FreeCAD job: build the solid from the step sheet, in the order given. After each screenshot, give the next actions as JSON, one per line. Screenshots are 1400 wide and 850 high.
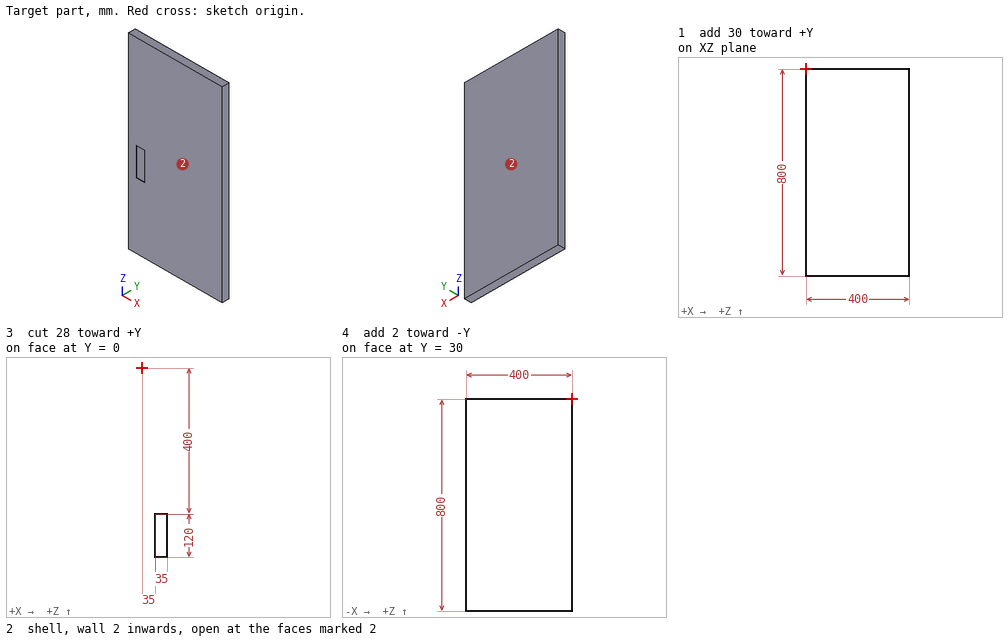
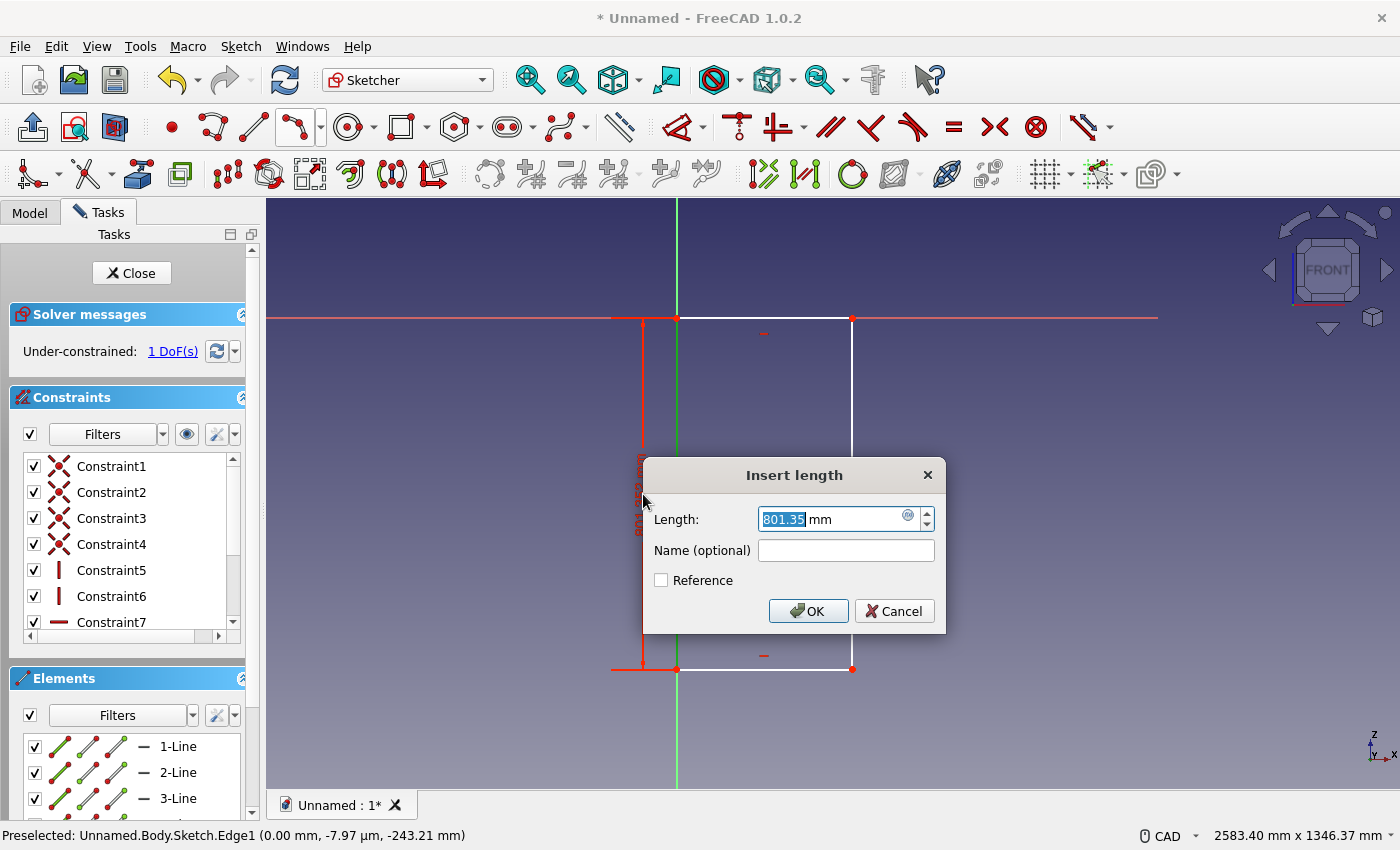
{"action": "type", "text": "800"}
{"action": "key", "text": "Return"}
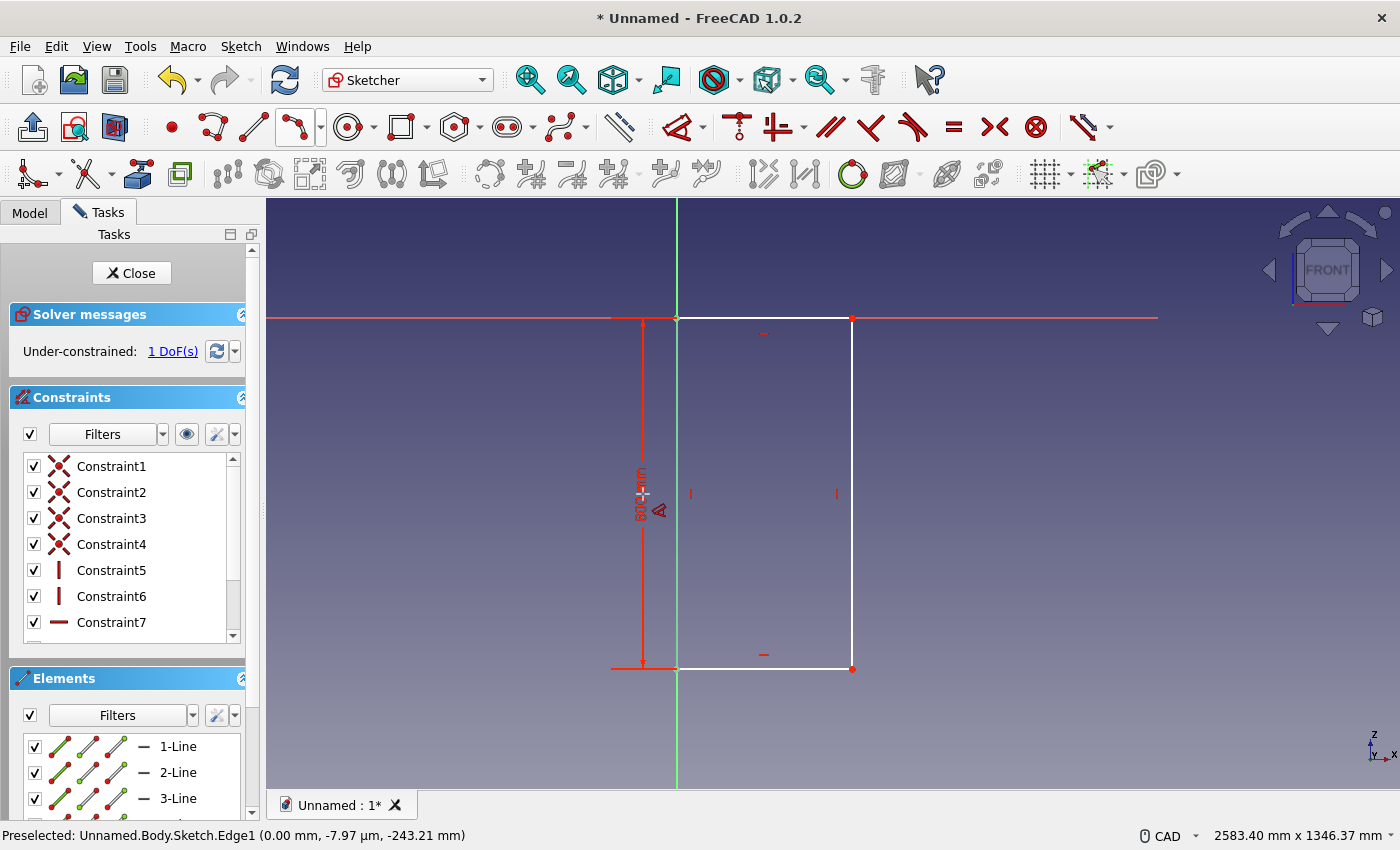
{"action": "left_click", "coordinate": [729, 669]}
{"action": "left_click", "coordinate": [764, 703]}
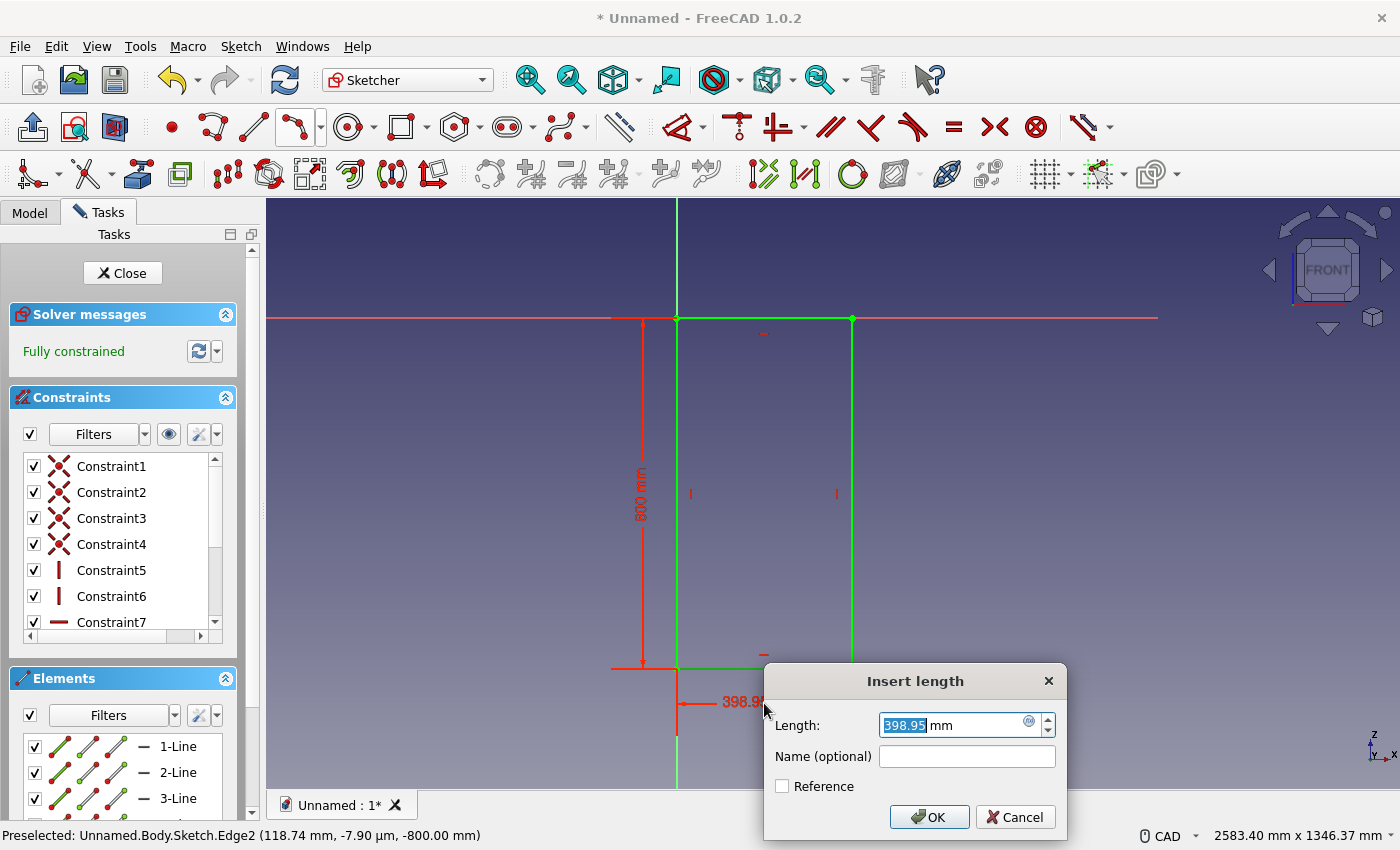
{"action": "type", "text": "400"}
{"action": "key", "text": "Return"}
{"action": "key", "text": "Escape"}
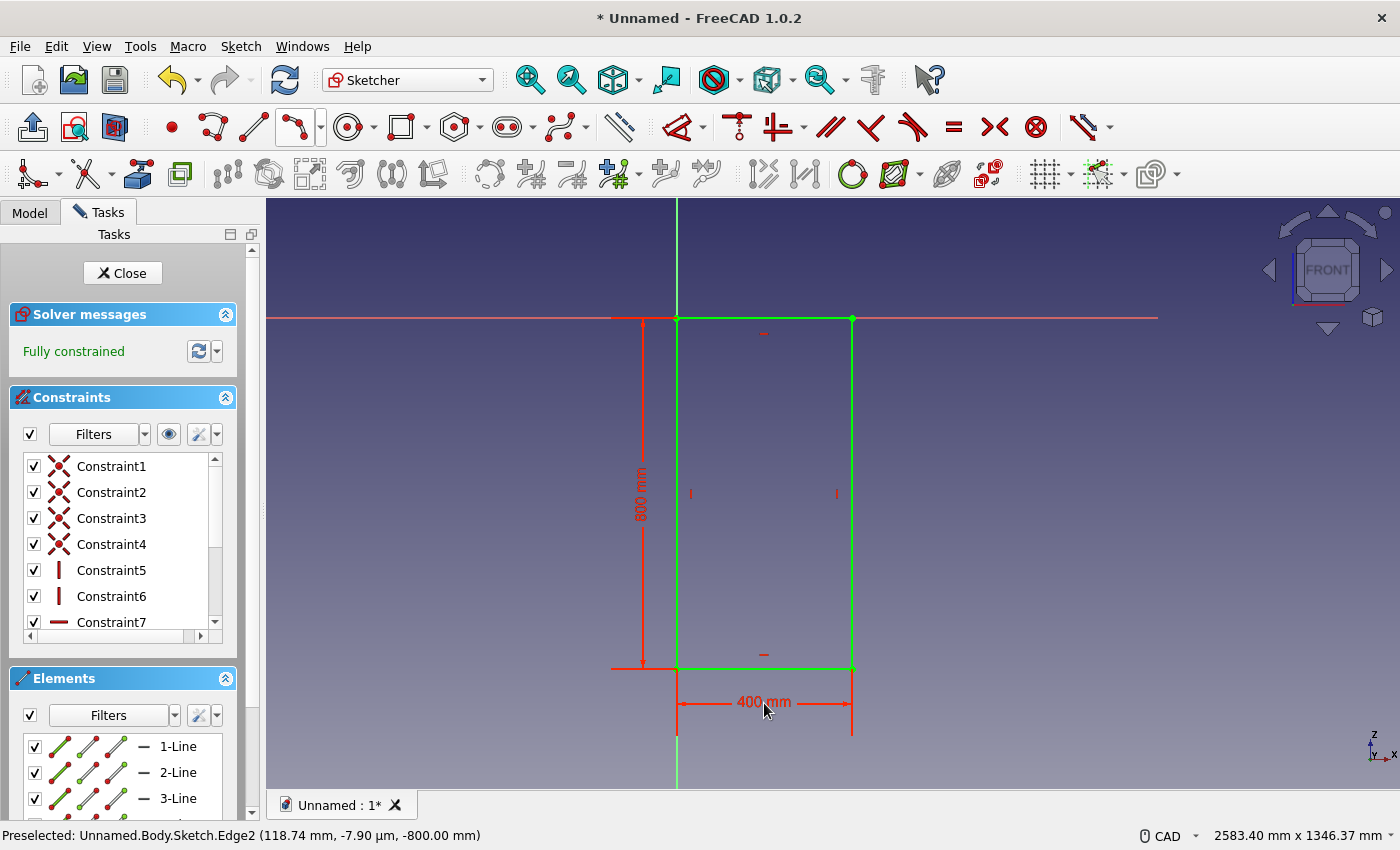
{"action": "left_click", "coordinate": [123, 273]}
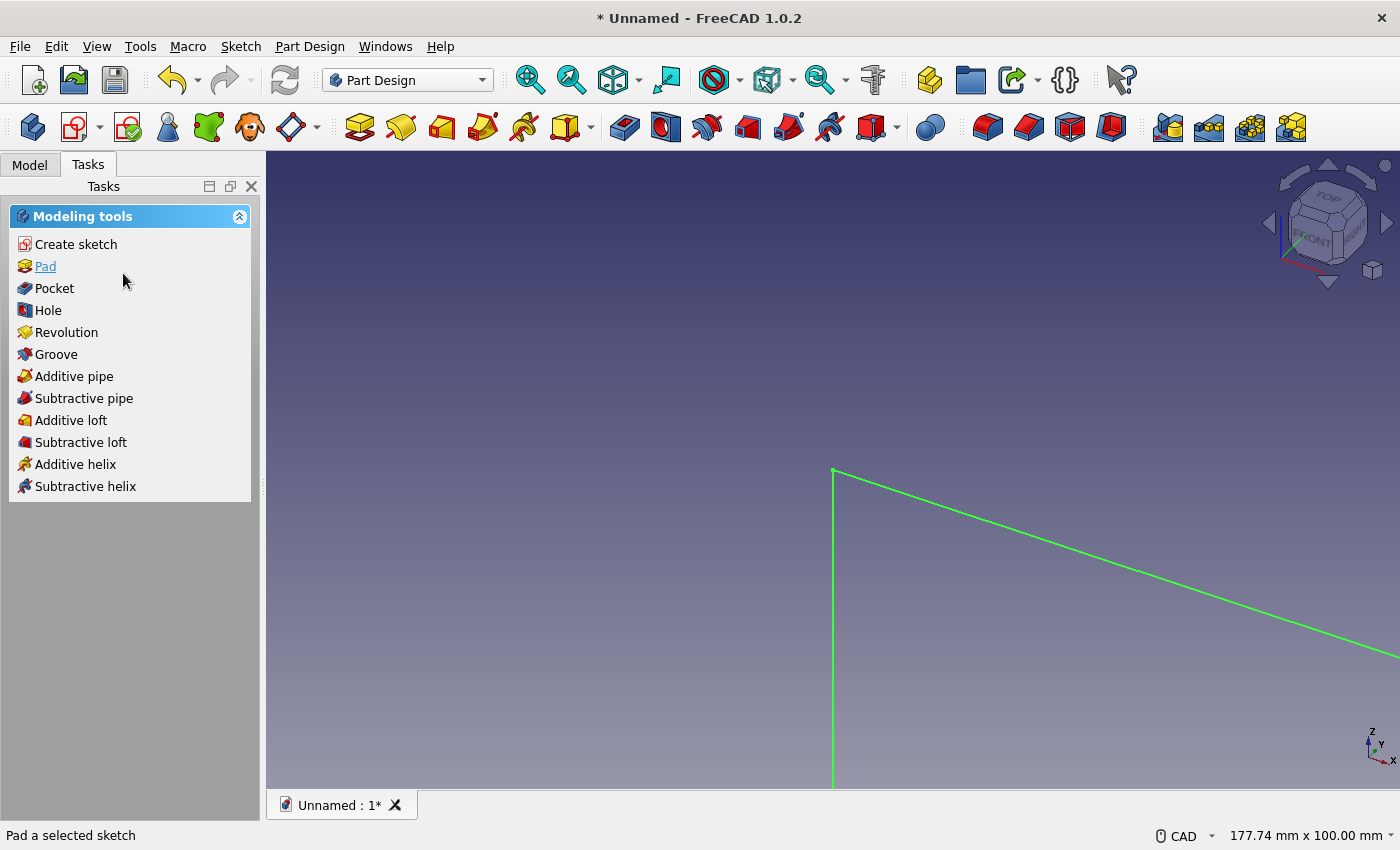
{"action": "left_click", "coordinate": [360, 128]}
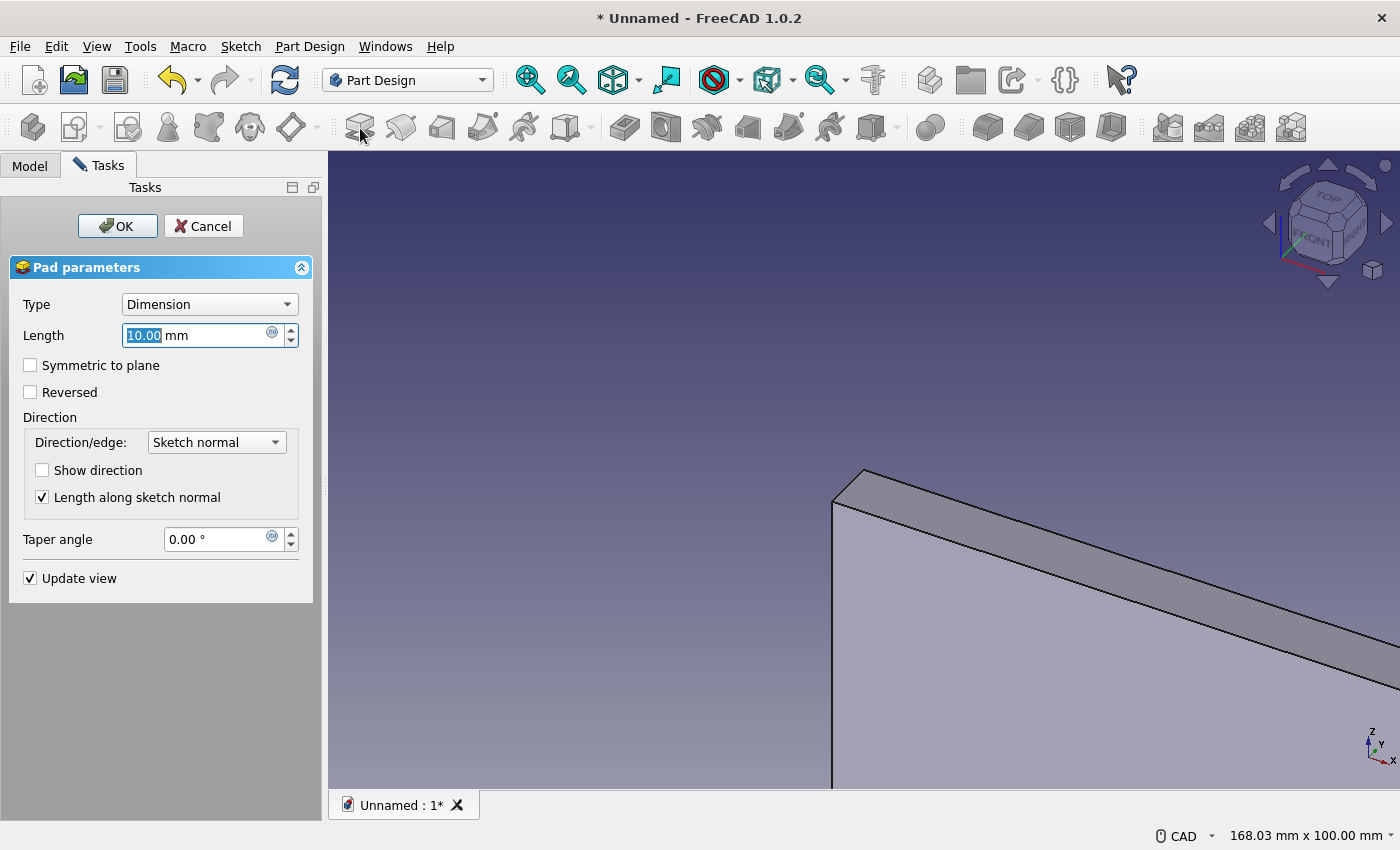
{"action": "type", "text": "30"}
{"action": "key", "text": "Tab"}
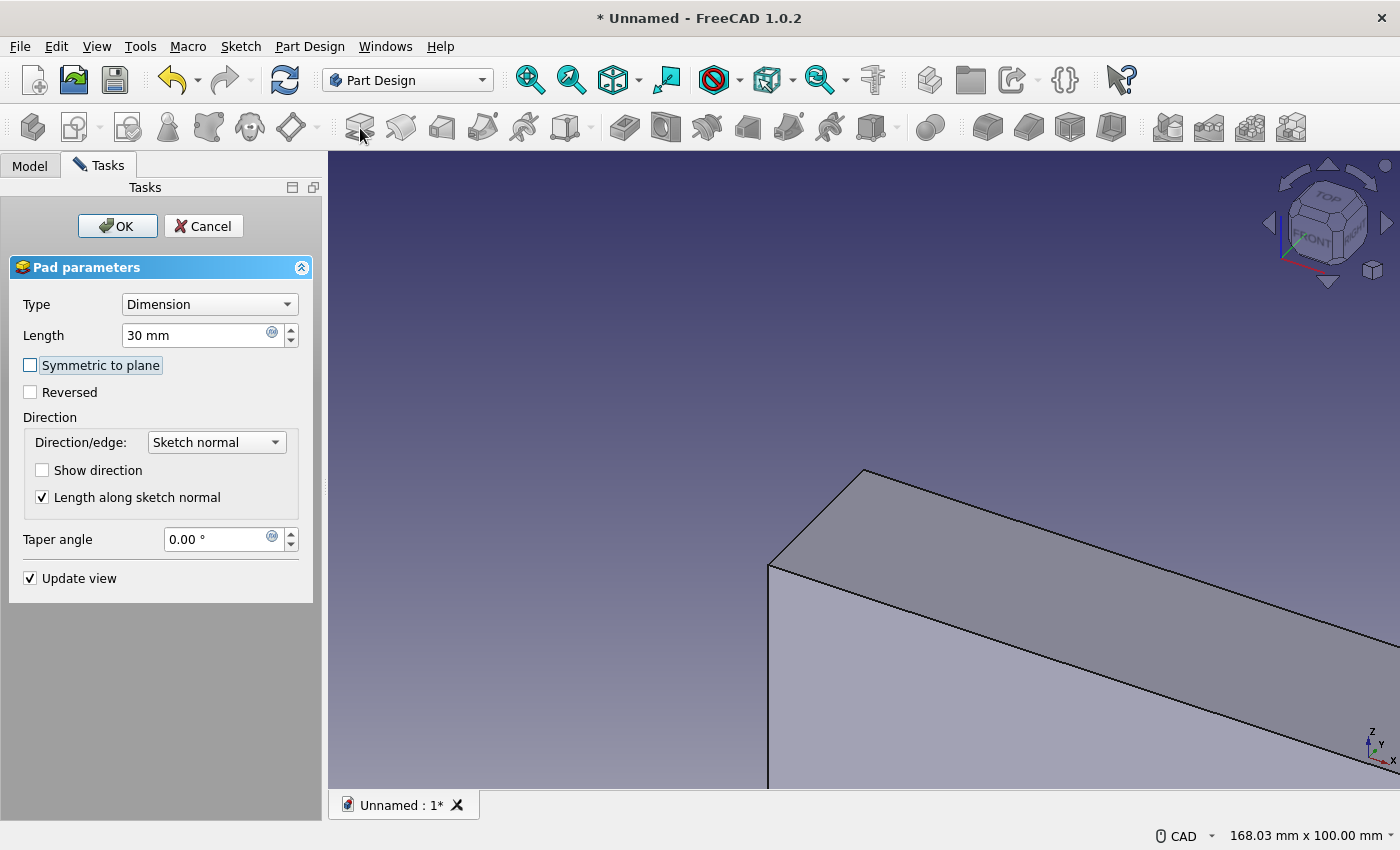
{"action": "left_click", "coordinate": [31, 392]}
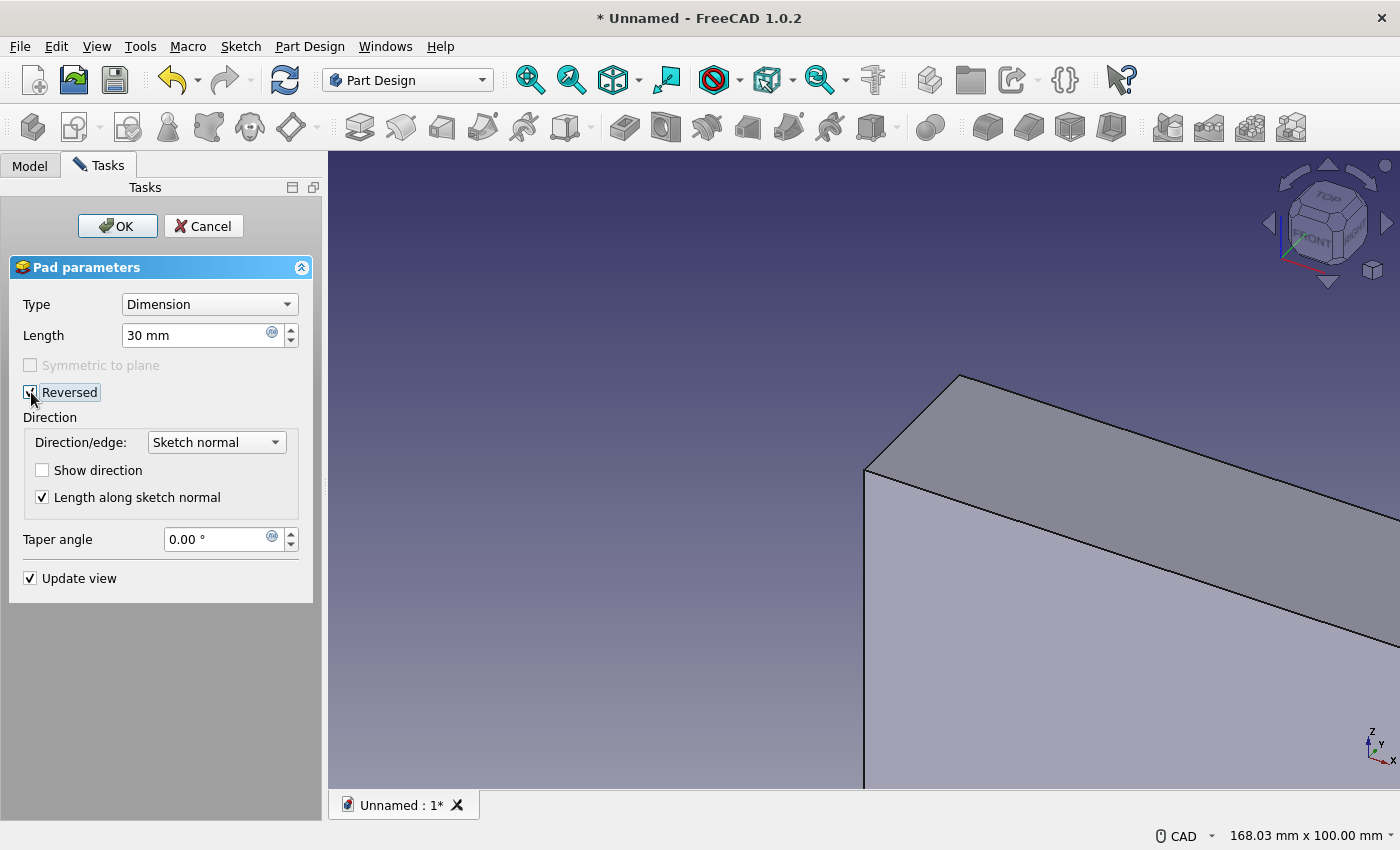
{"action": "left_click", "coordinate": [118, 226]}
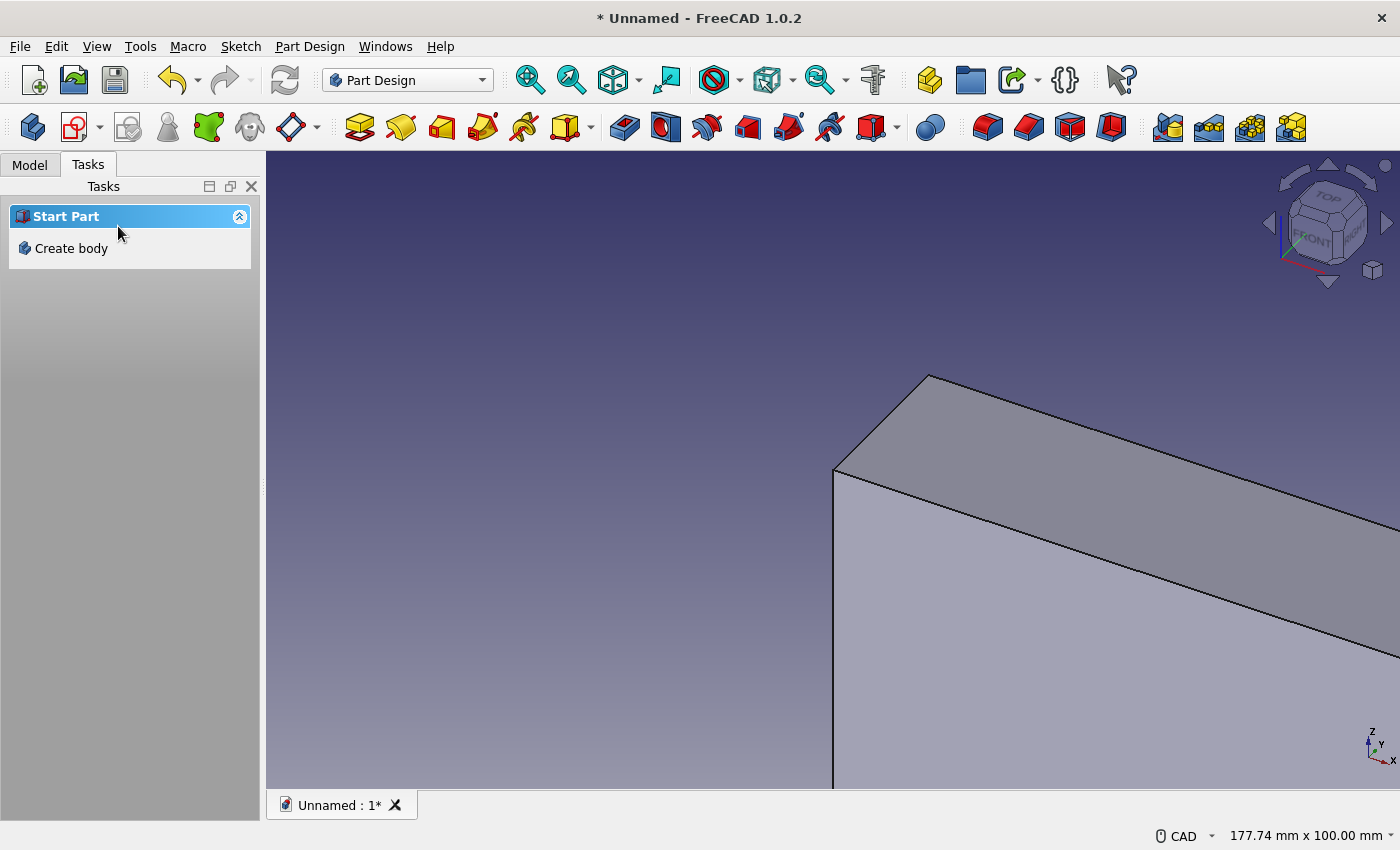
{"action": "left_click", "coordinate": [531, 80]}